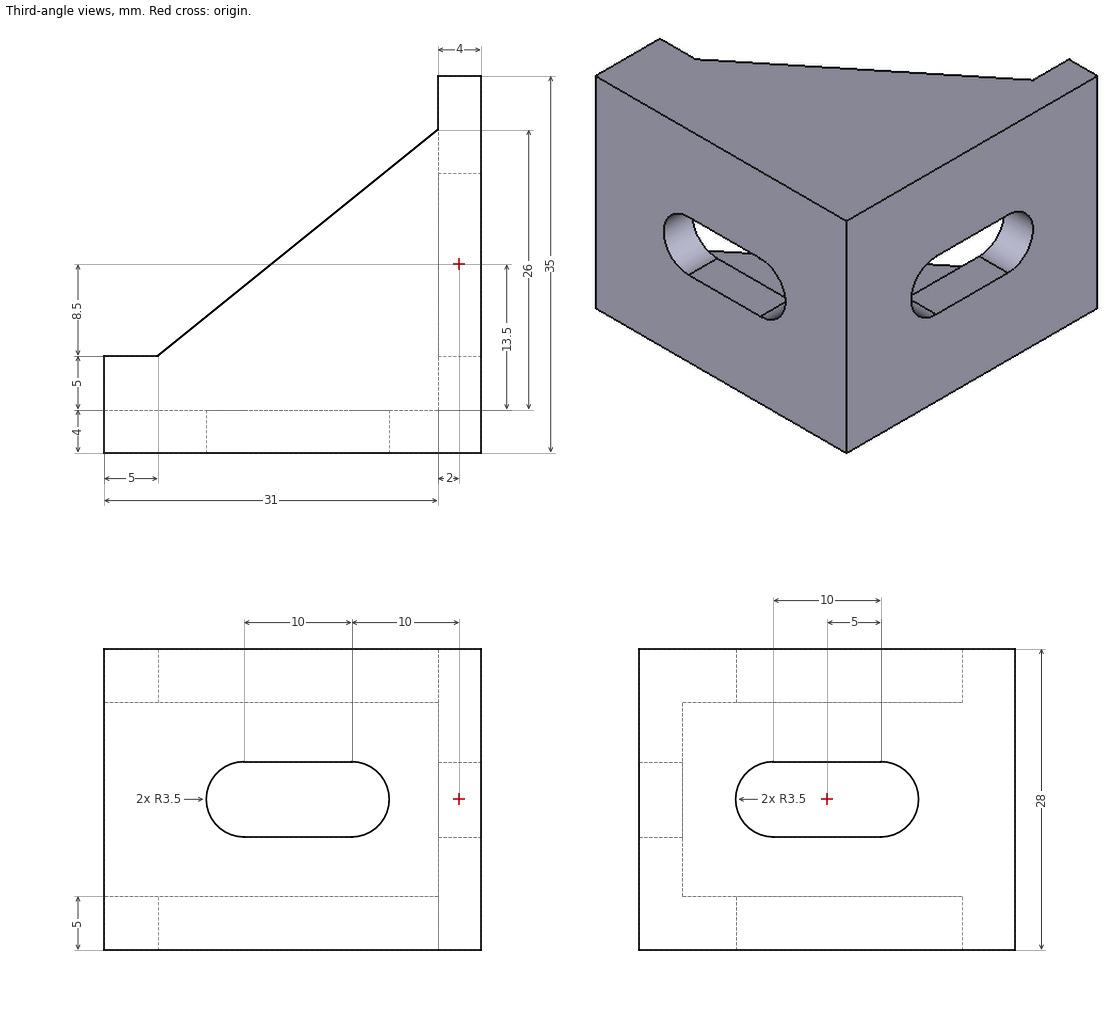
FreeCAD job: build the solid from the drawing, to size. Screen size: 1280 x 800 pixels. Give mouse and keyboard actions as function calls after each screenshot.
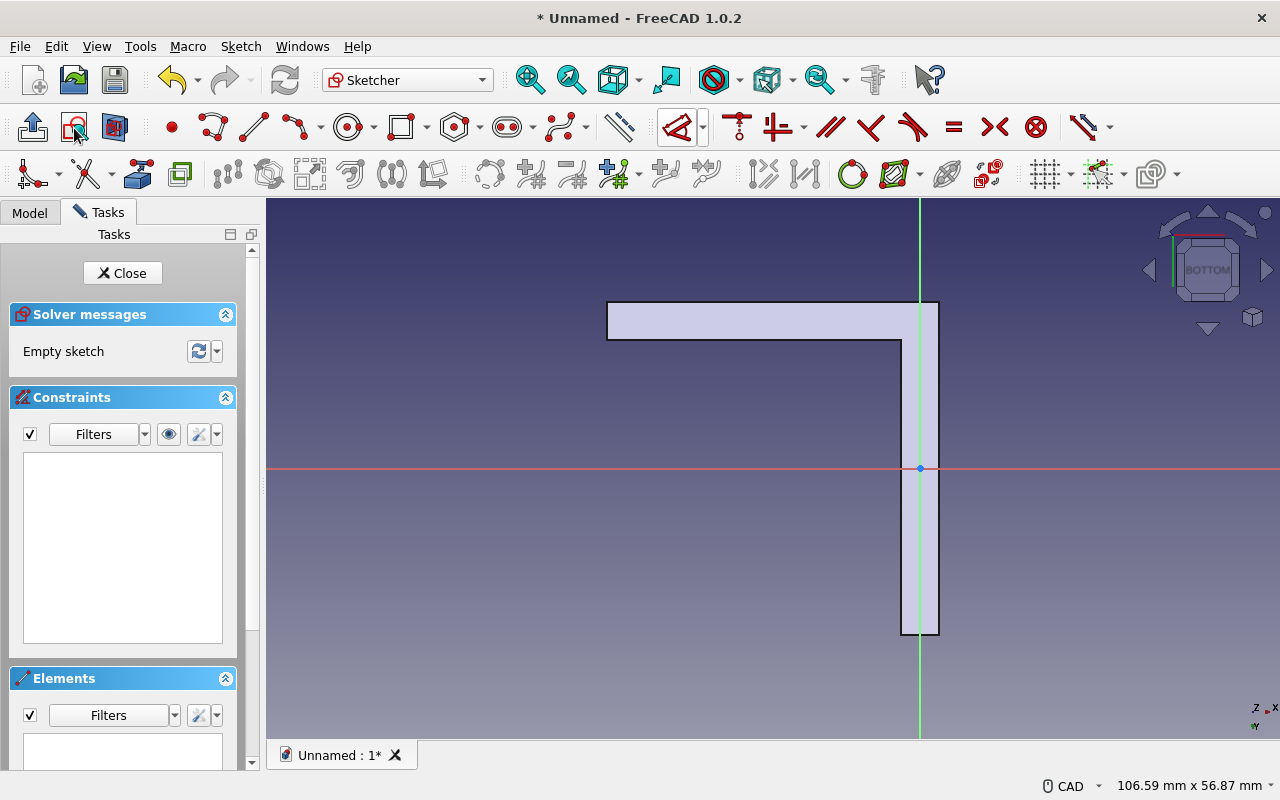
scroll(883, 454, up, 2)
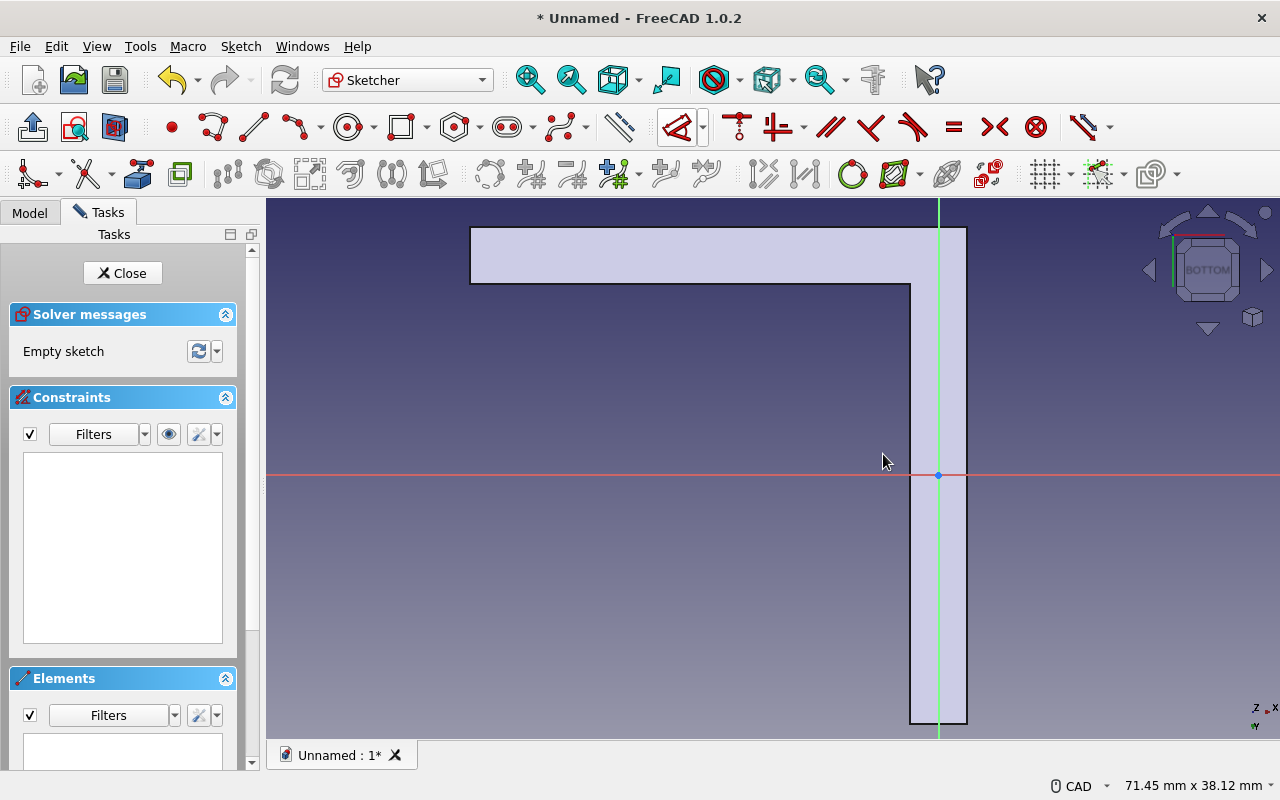
click(213, 128)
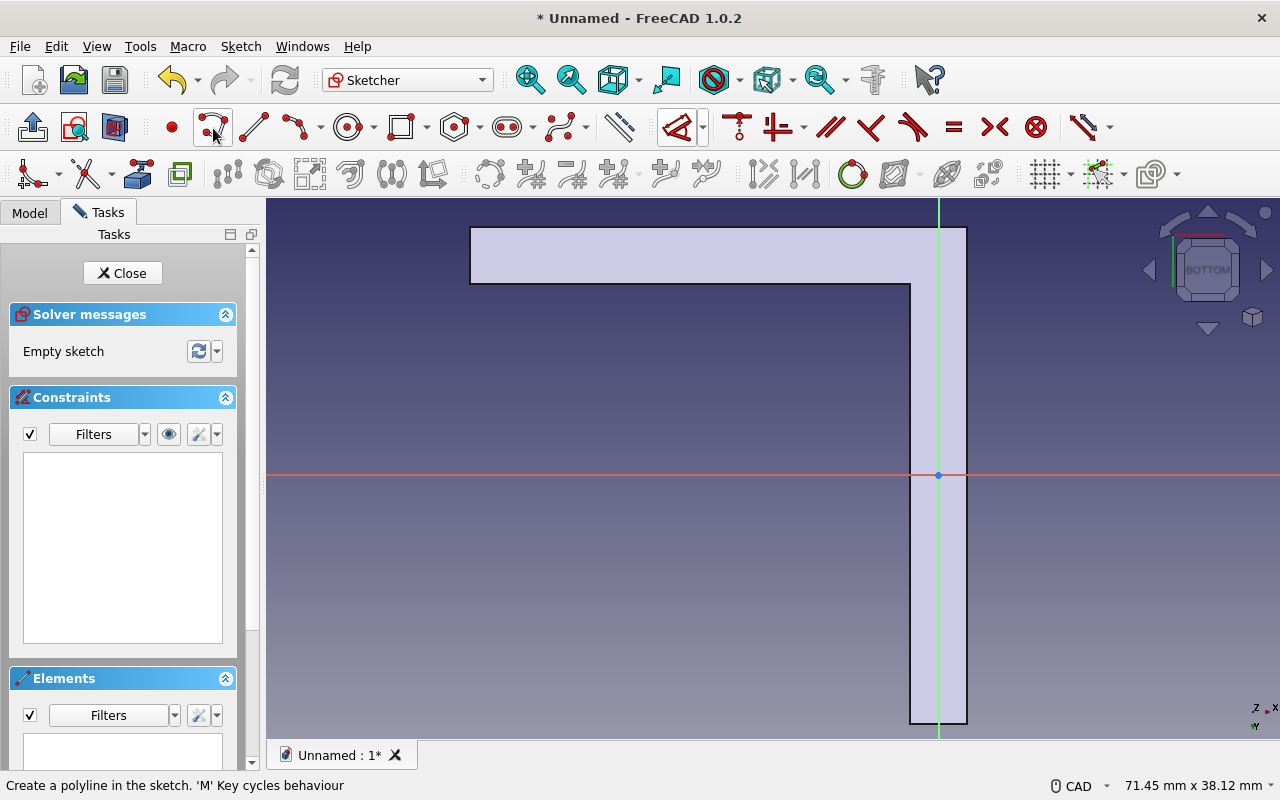
click(910, 653)
click(910, 284)
click(470, 284)
click(470, 355)
click(541, 355)
click(910, 654)
key(Escape)
key(Escape)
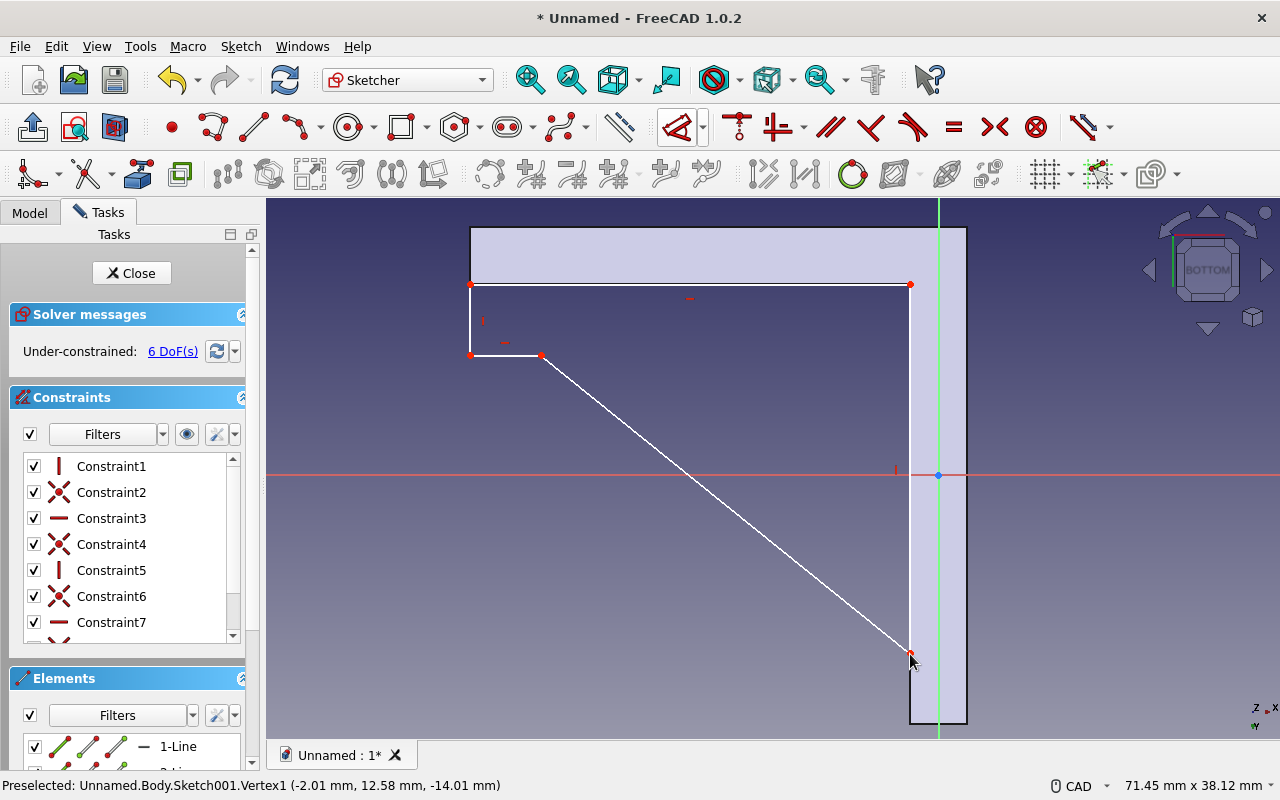
click(470, 306)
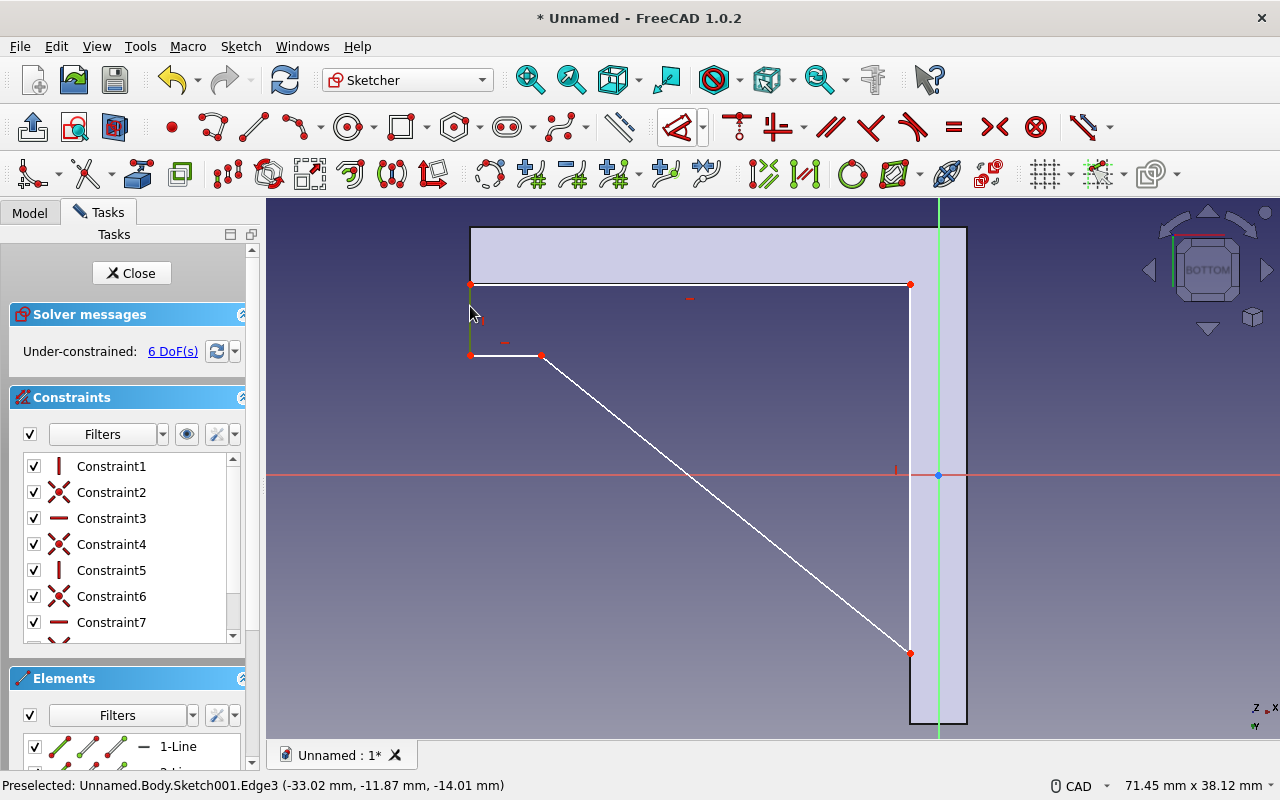
click(702, 128)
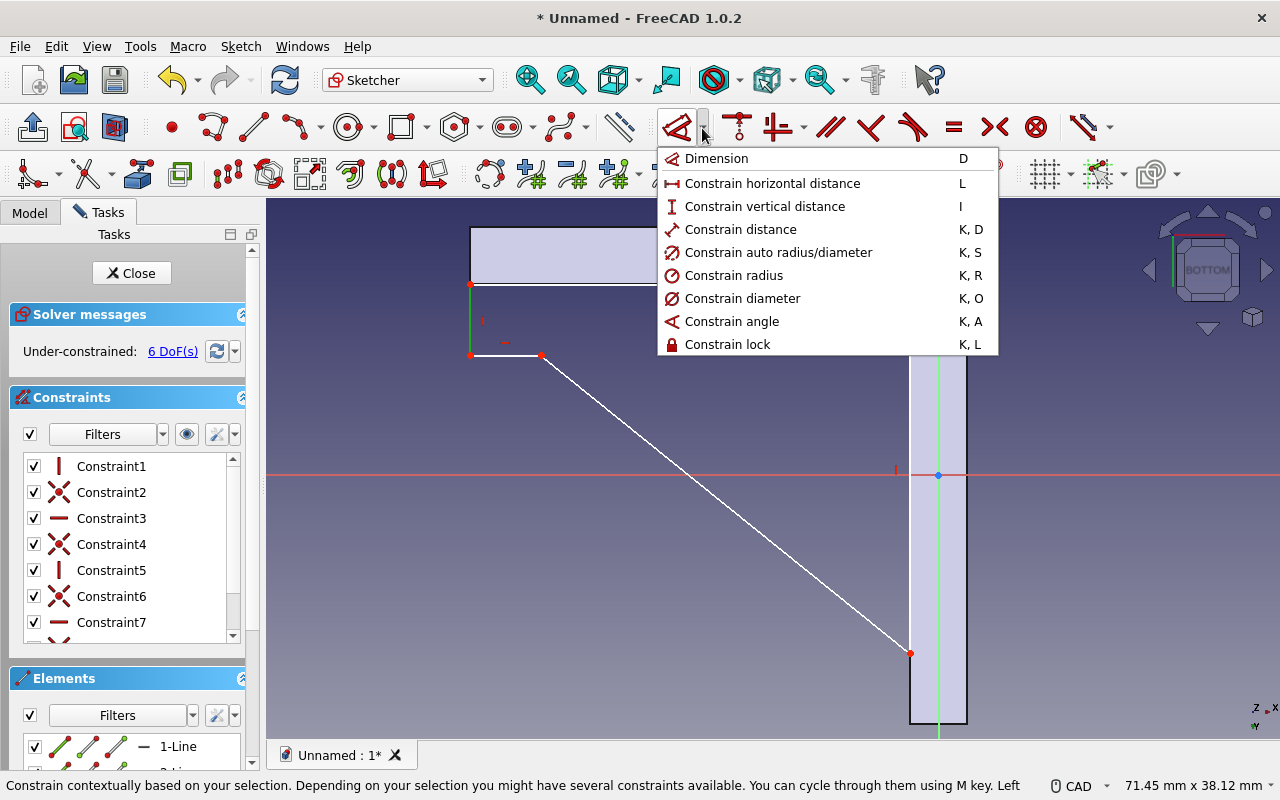
click(828, 206)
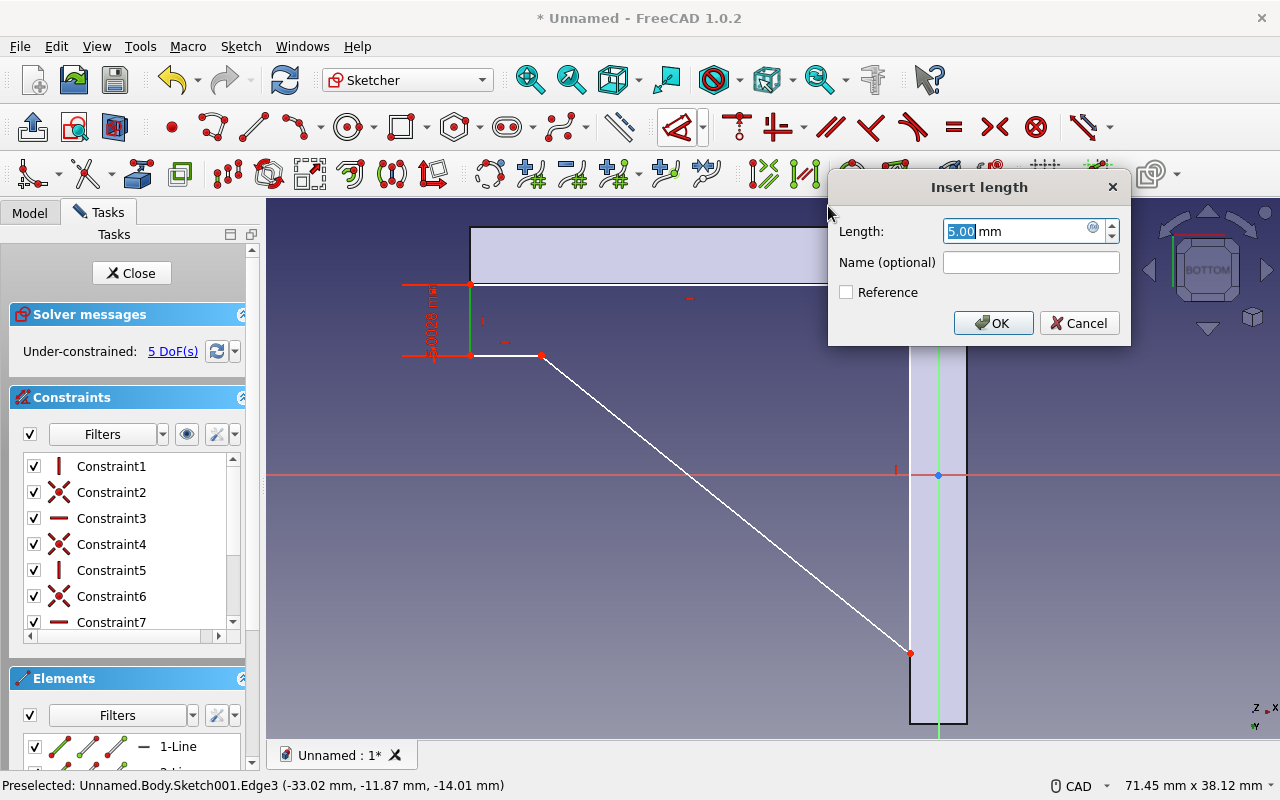
text(5)
key(Return)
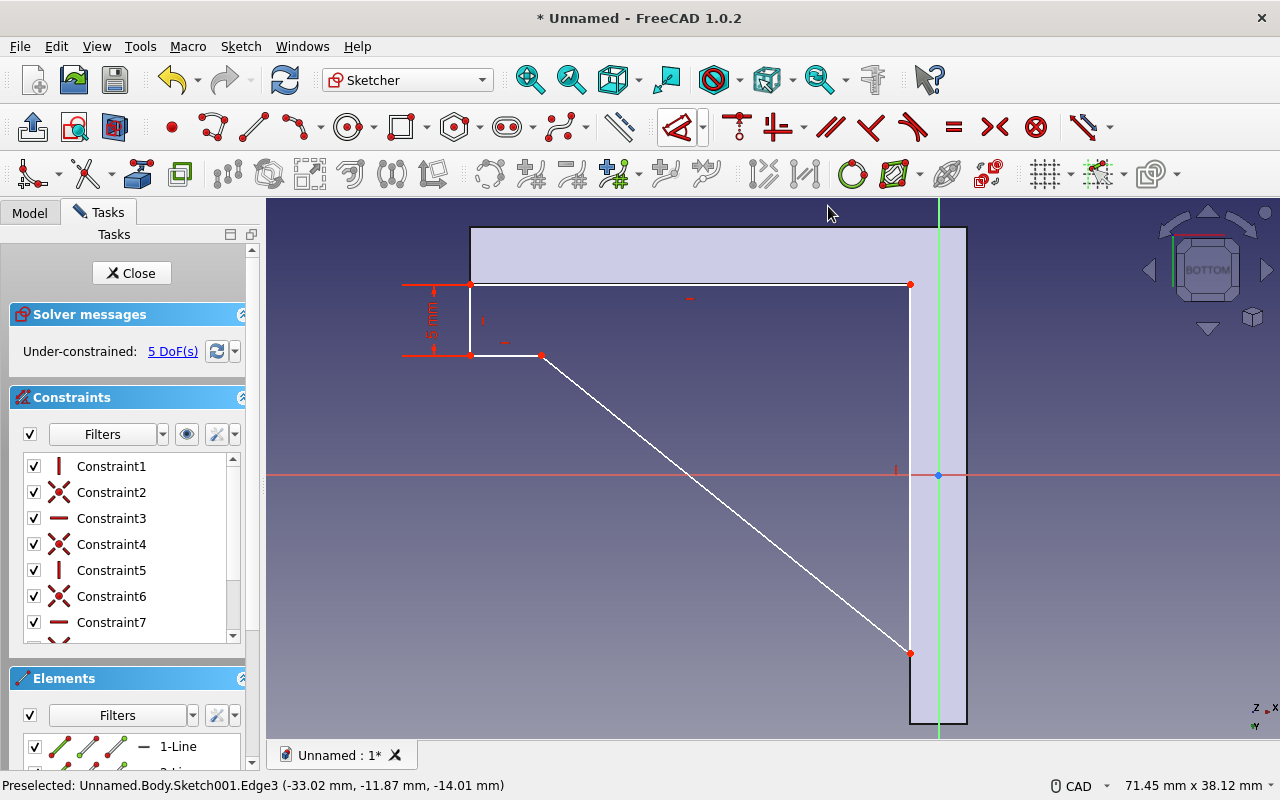
click(491, 356)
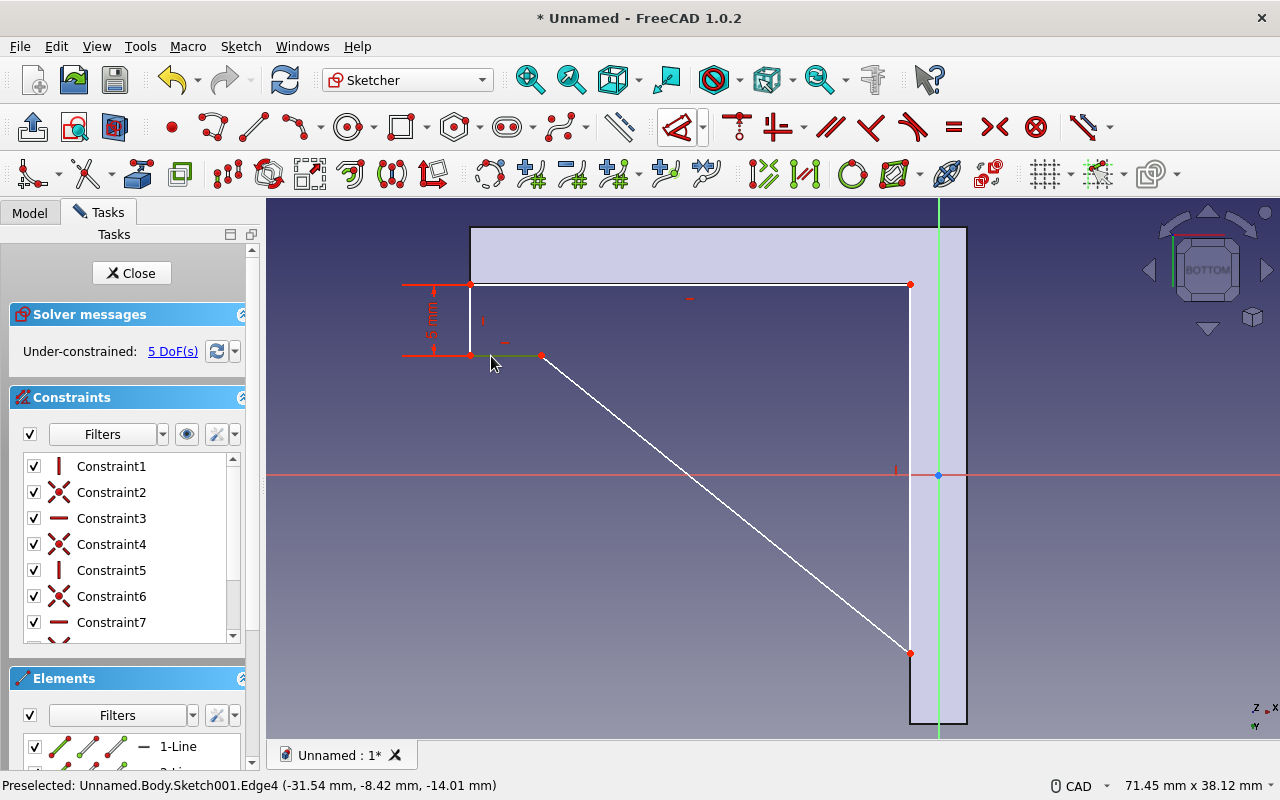
key(l)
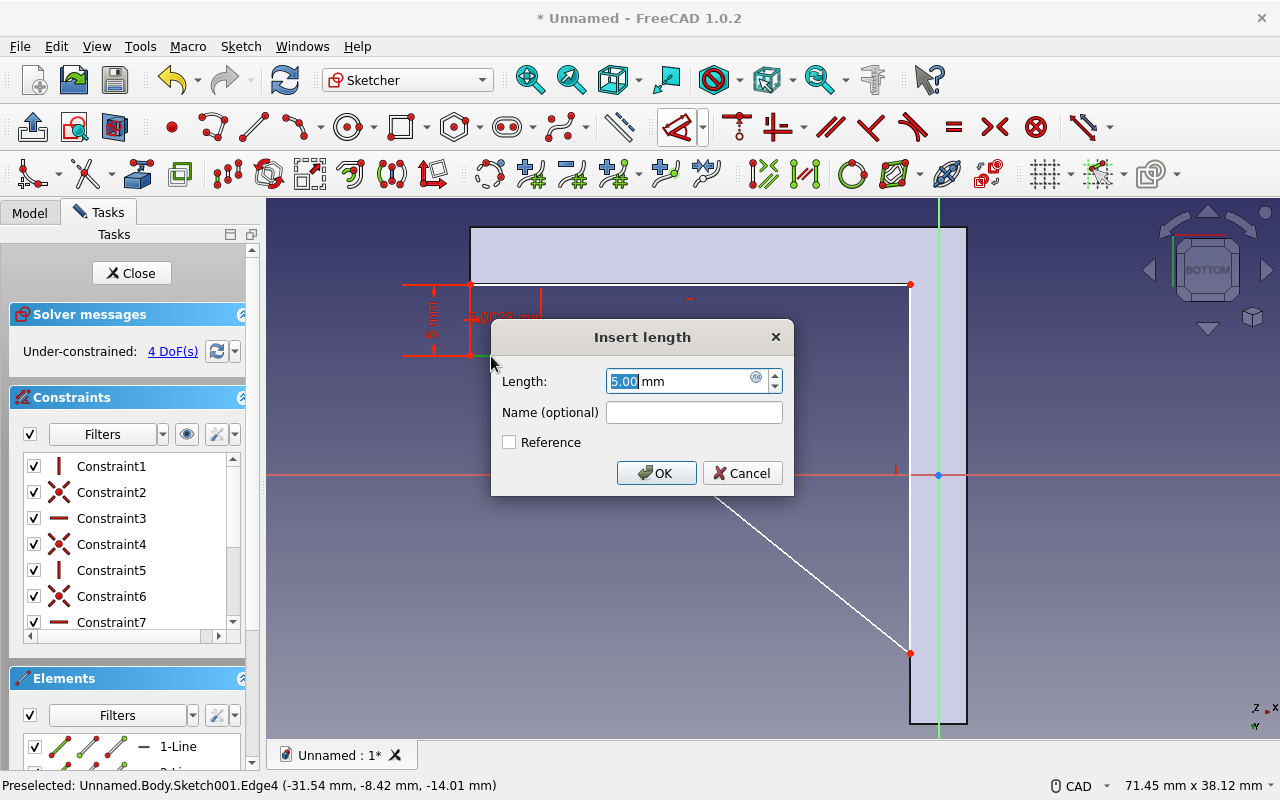
text(5)
key(Return)